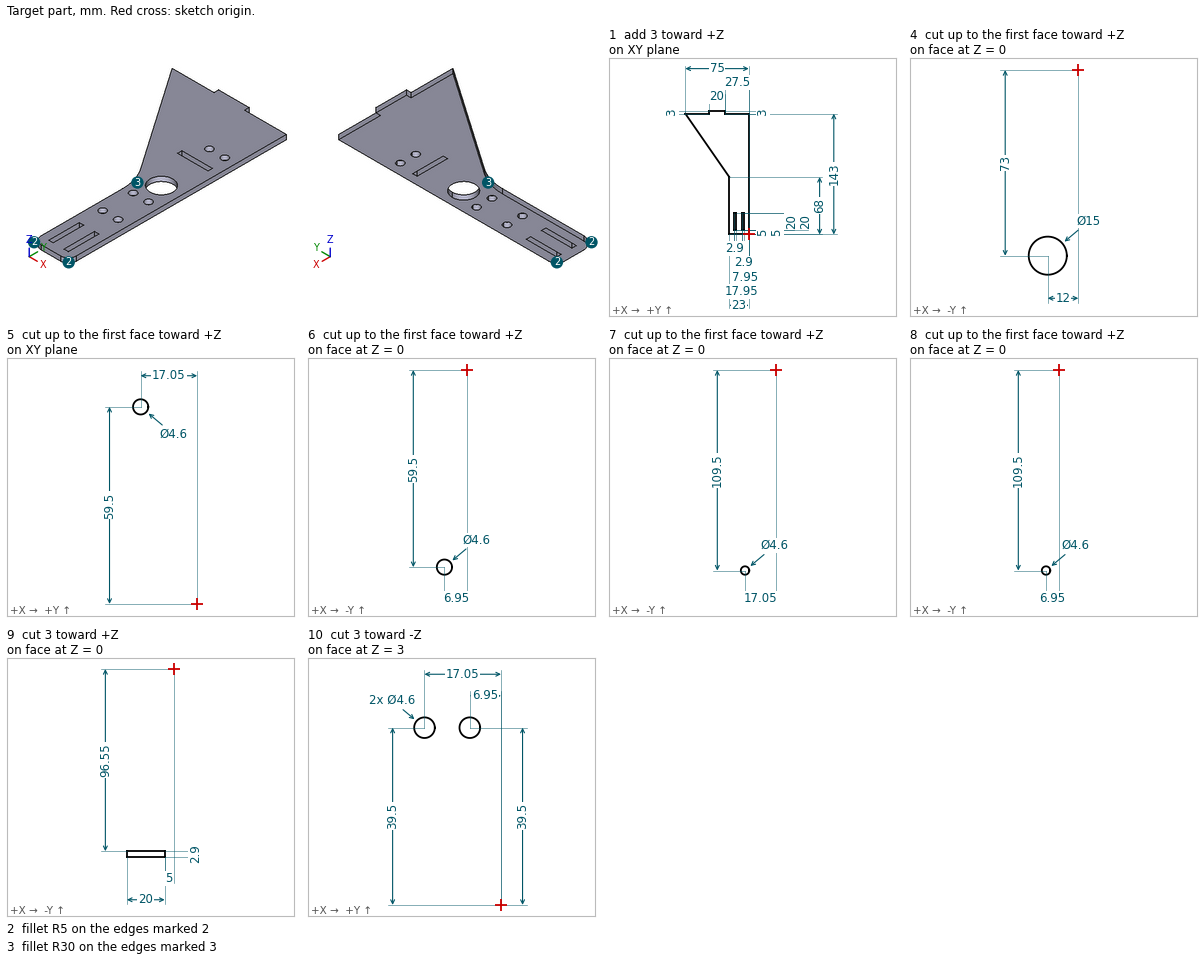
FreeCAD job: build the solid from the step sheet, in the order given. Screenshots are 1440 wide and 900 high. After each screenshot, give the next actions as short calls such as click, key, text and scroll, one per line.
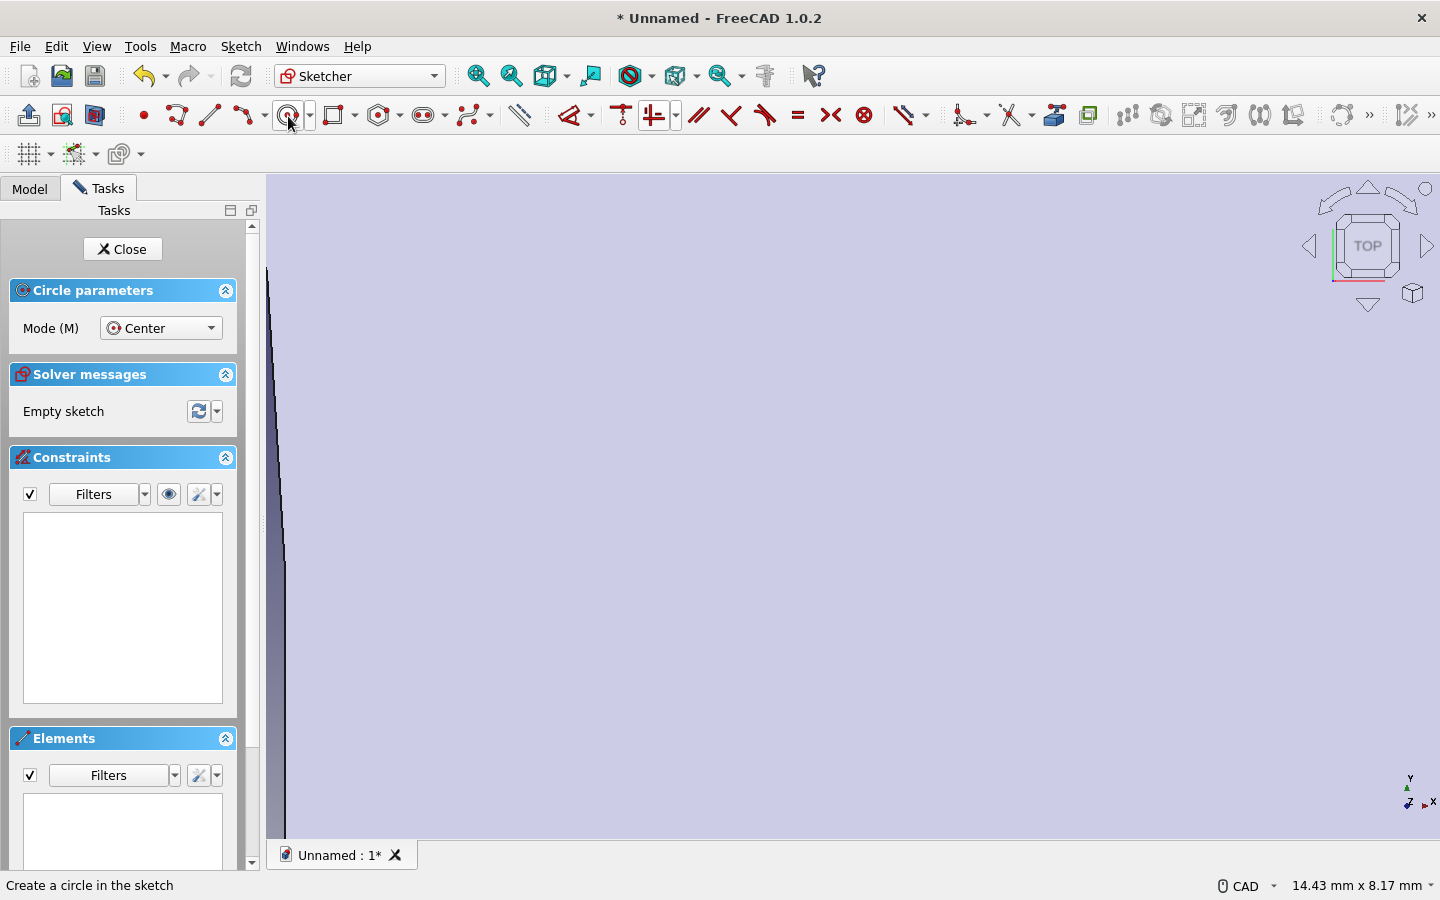
click(769, 496)
move(901, 364)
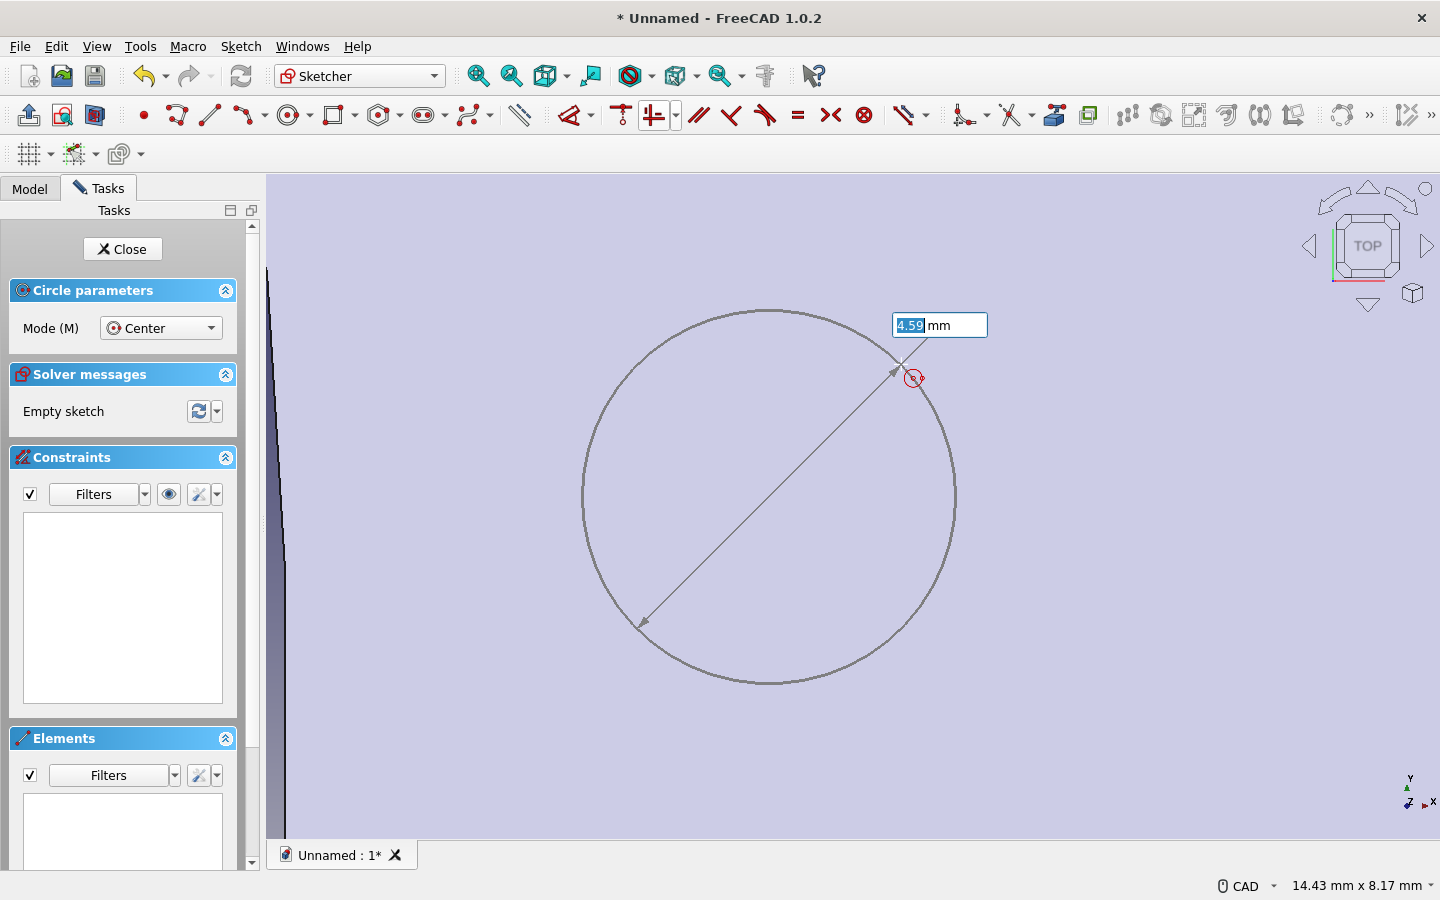
text(4.6)
key(Return)
key(Escape)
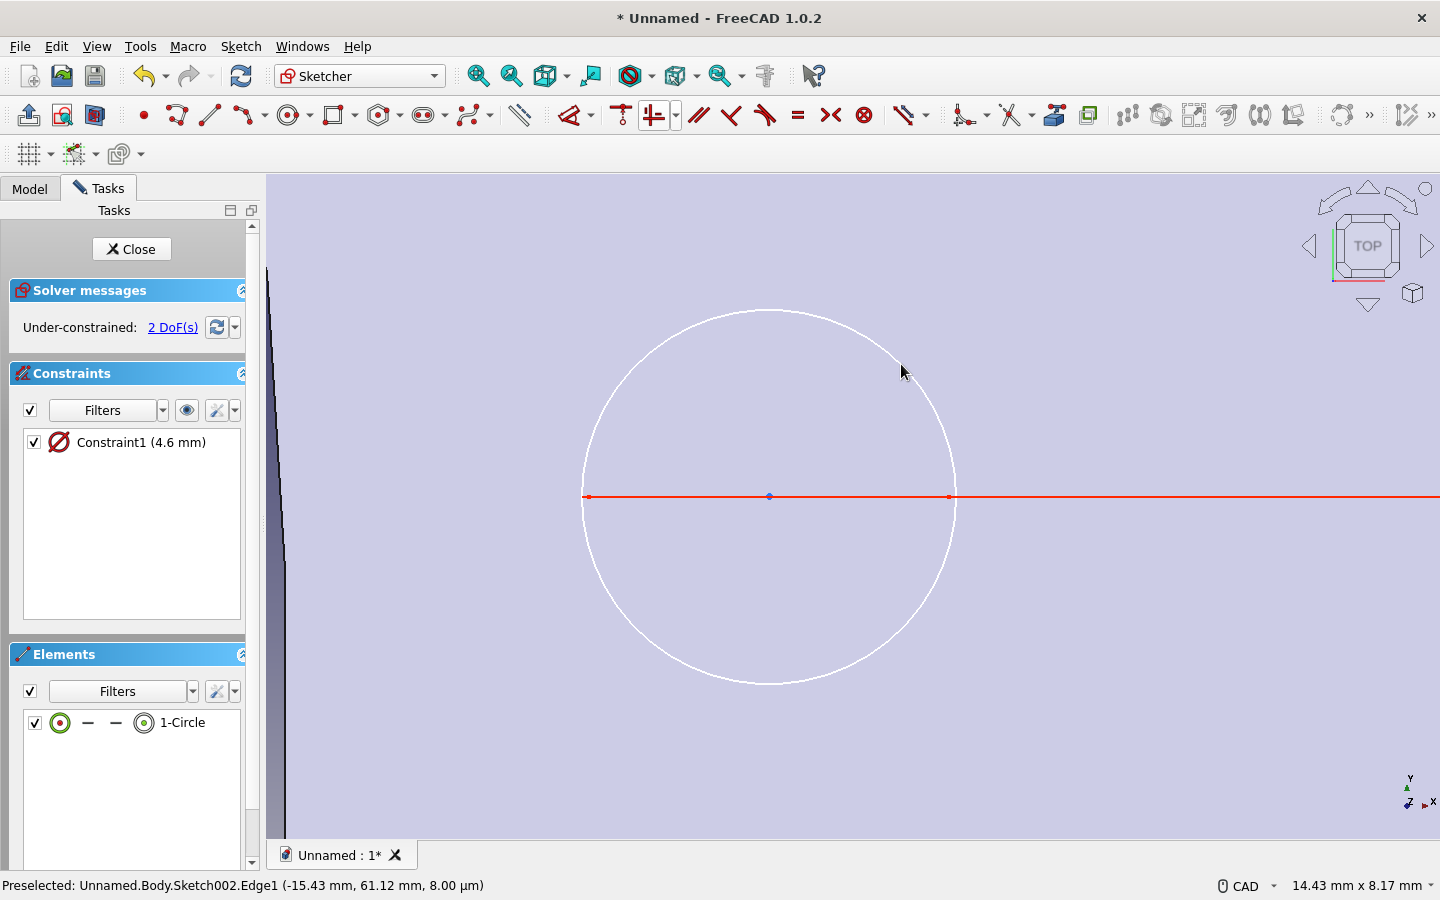
key(d)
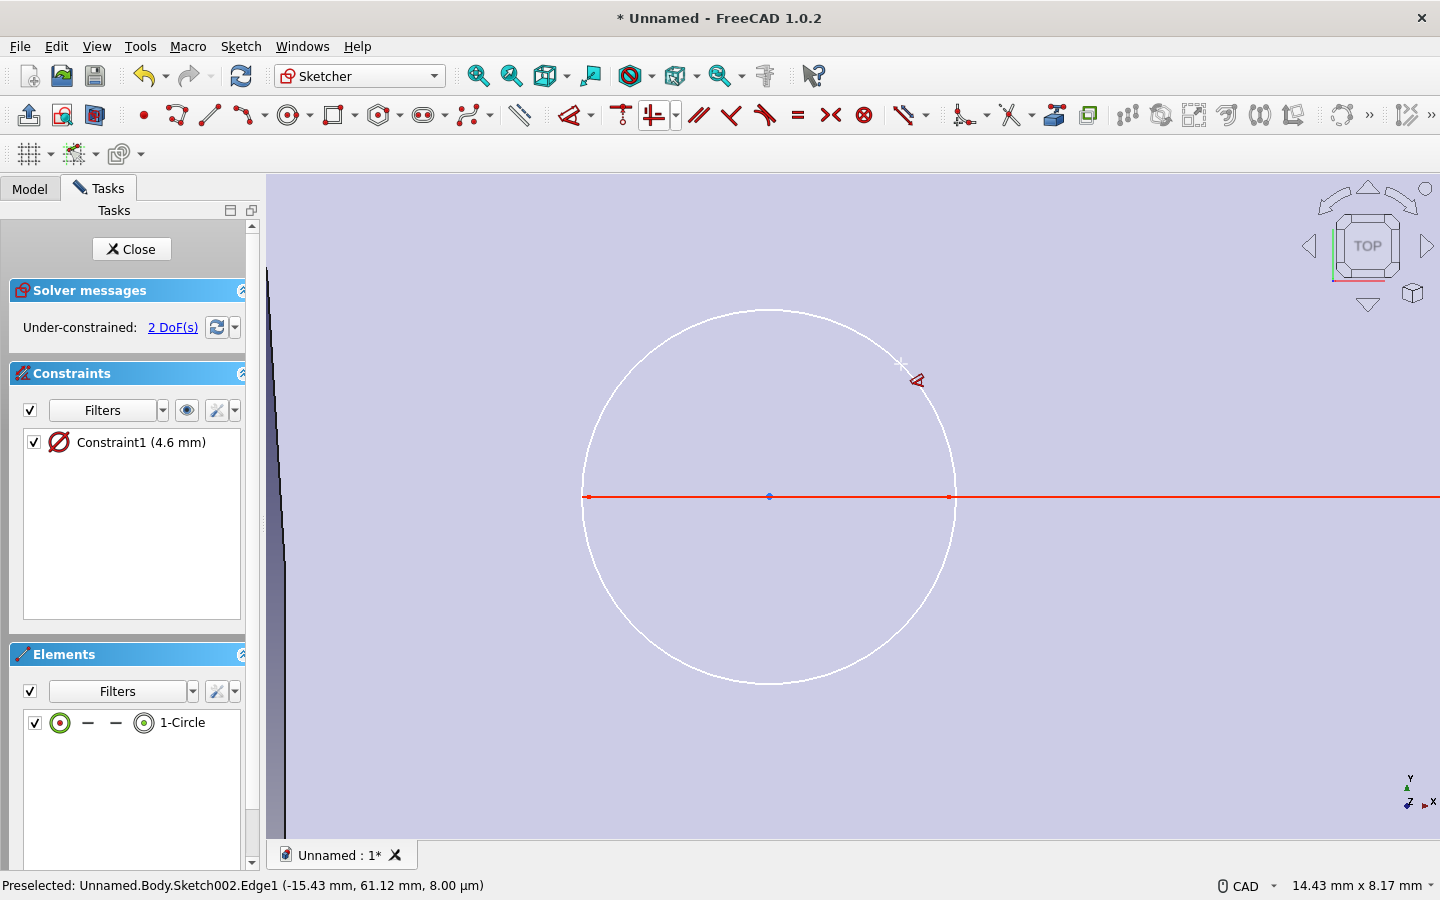
click(769, 497)
click(735, 654)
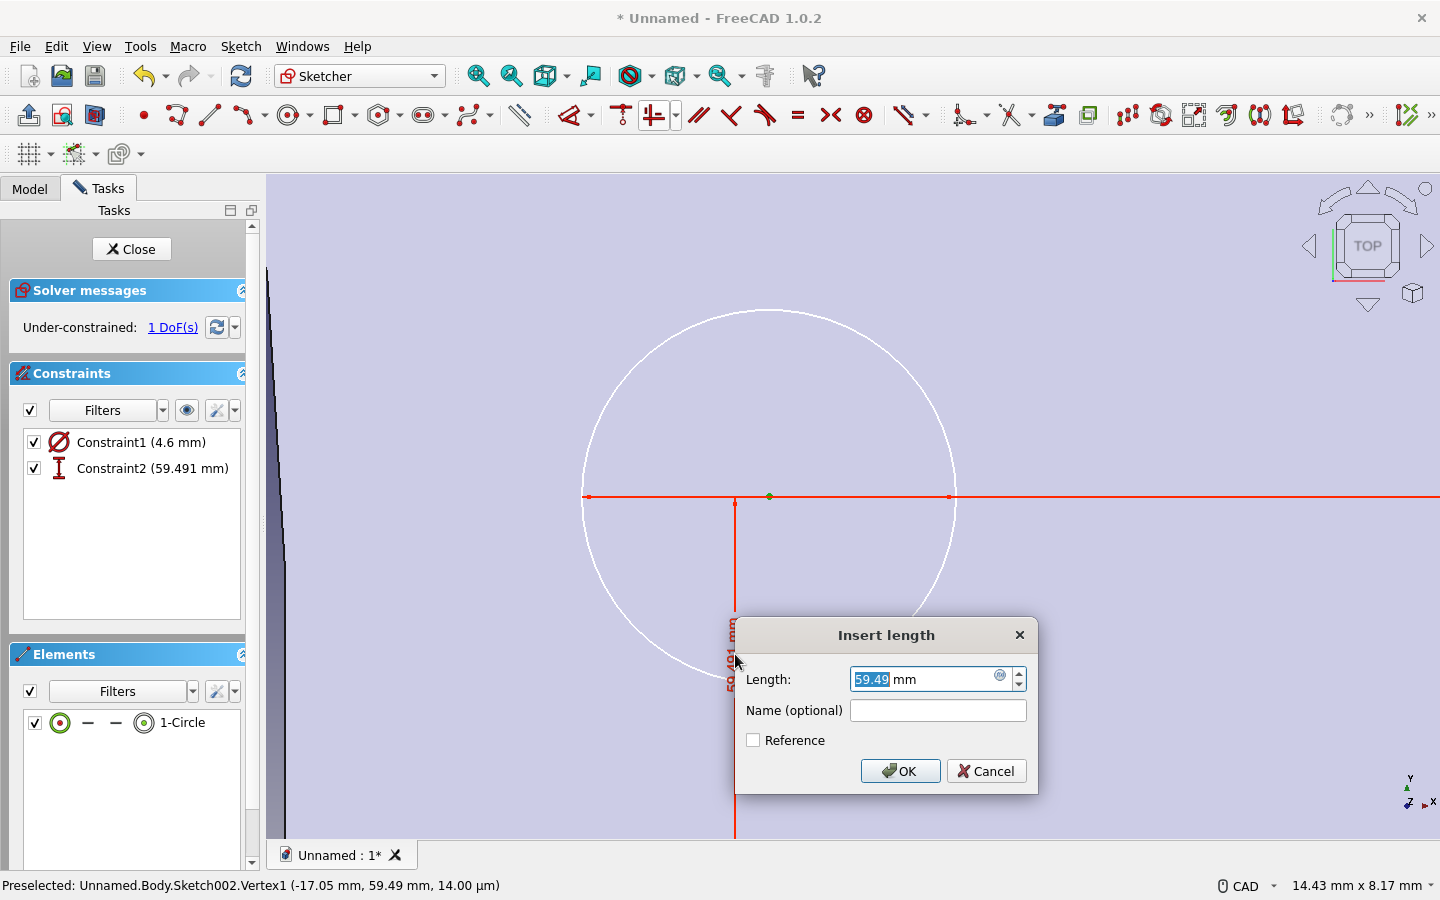
text(59.5)
key(Return)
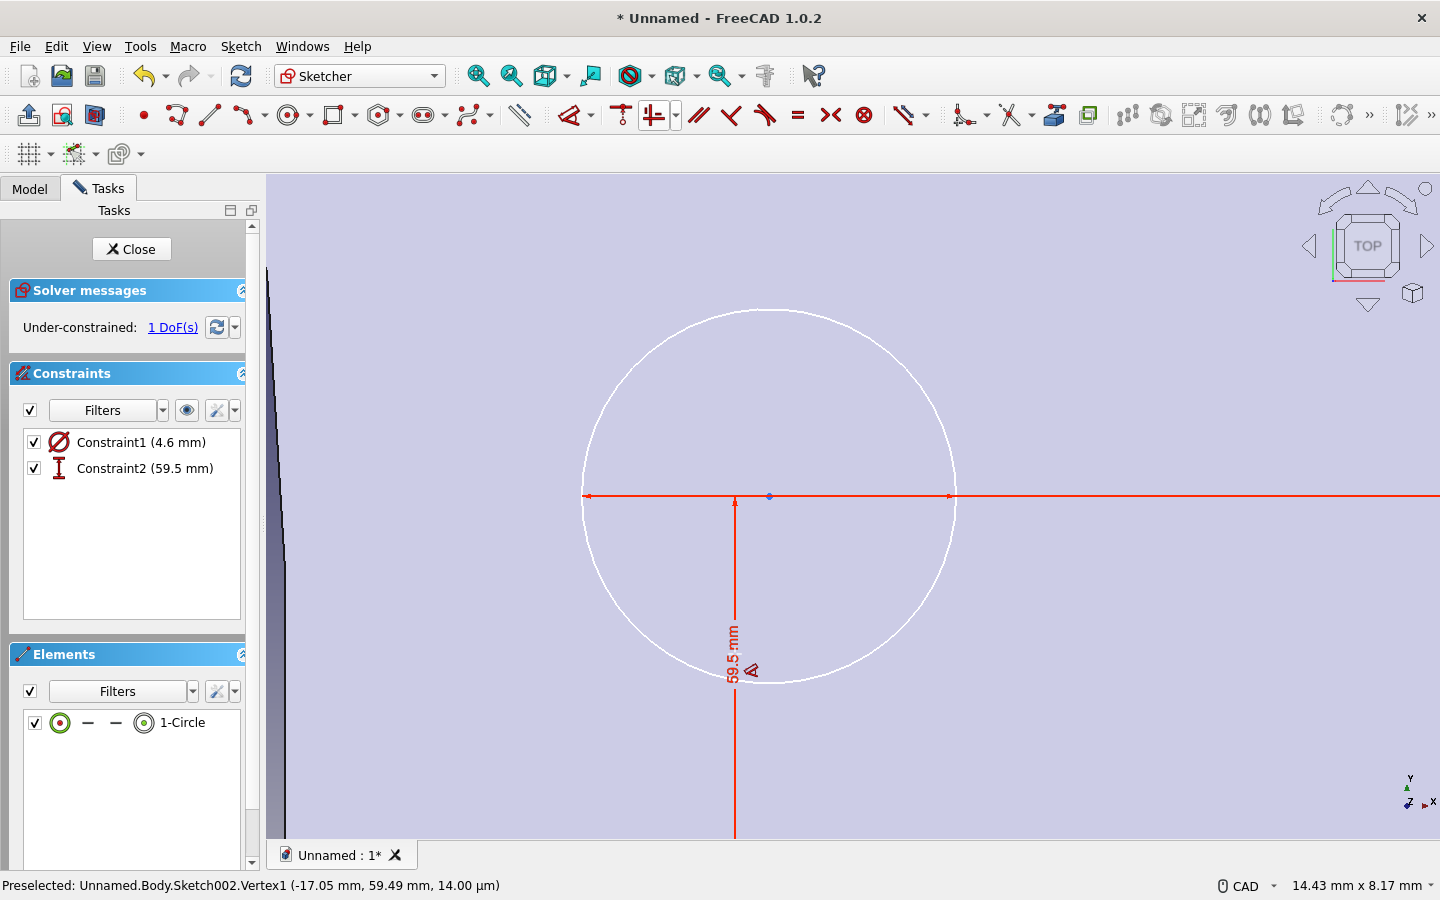
click(769, 496)
click(1022, 462)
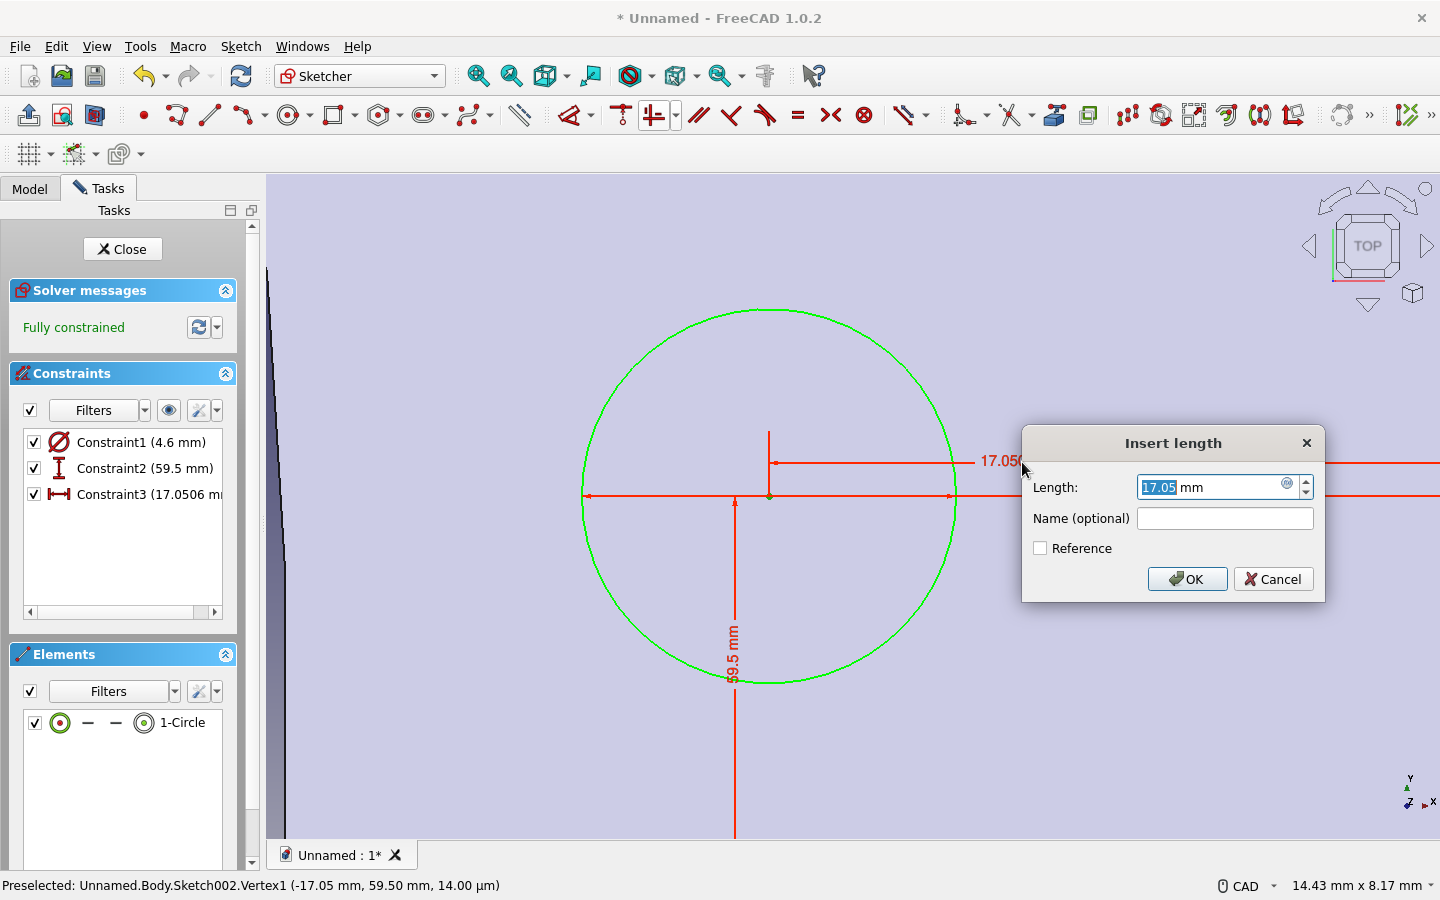
text(17.05)
key(Return)
key(Escape)